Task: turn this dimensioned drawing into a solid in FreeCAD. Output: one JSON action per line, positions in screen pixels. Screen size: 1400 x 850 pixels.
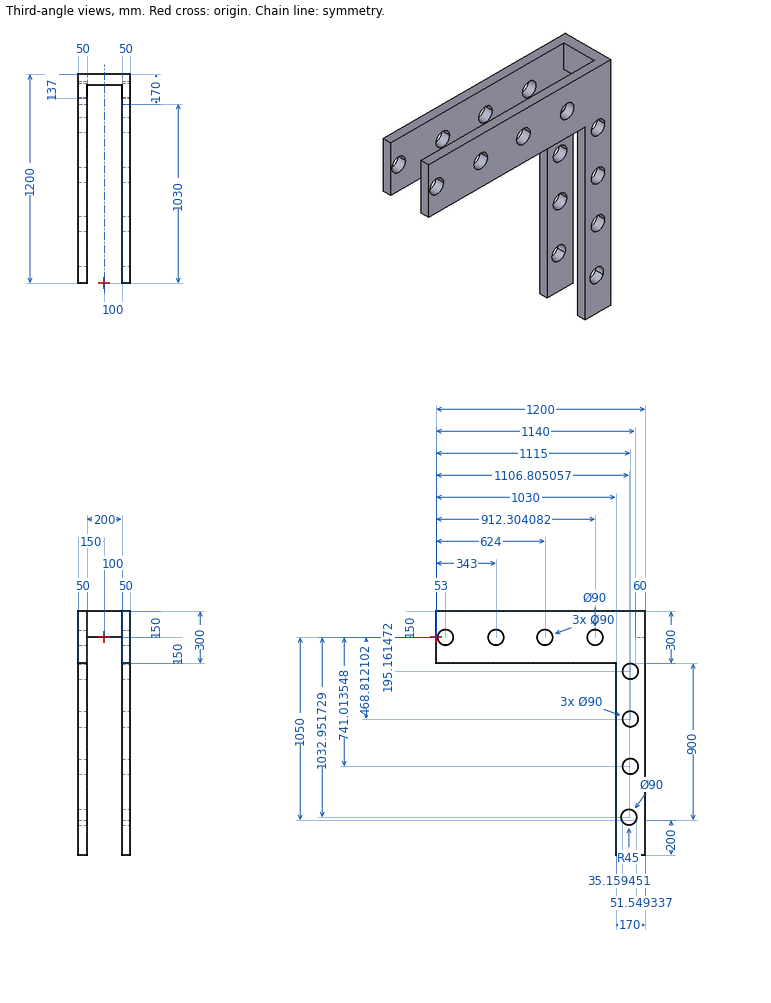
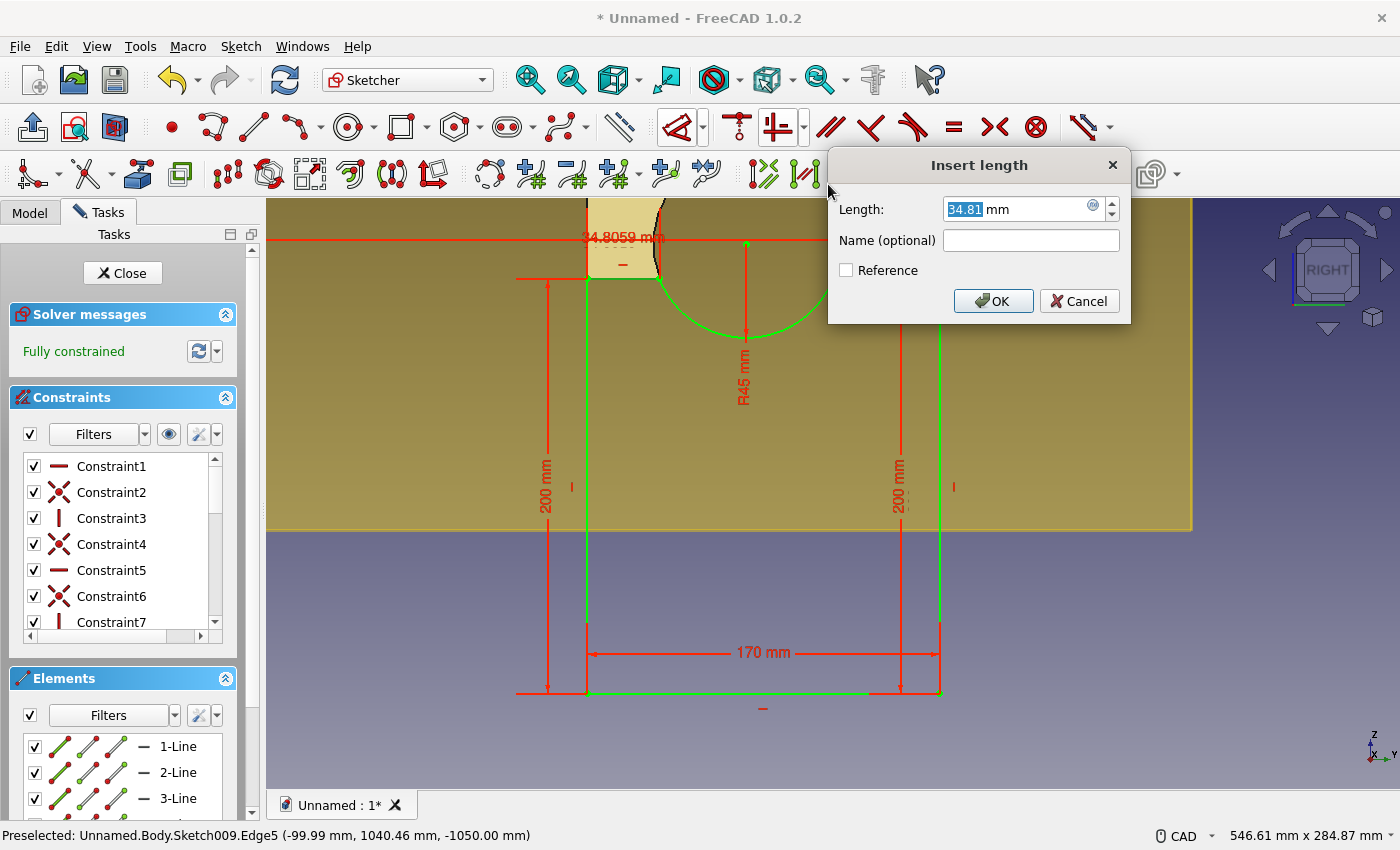
{"action": "type", "text": "35.159451"}
{"action": "key", "text": "Return"}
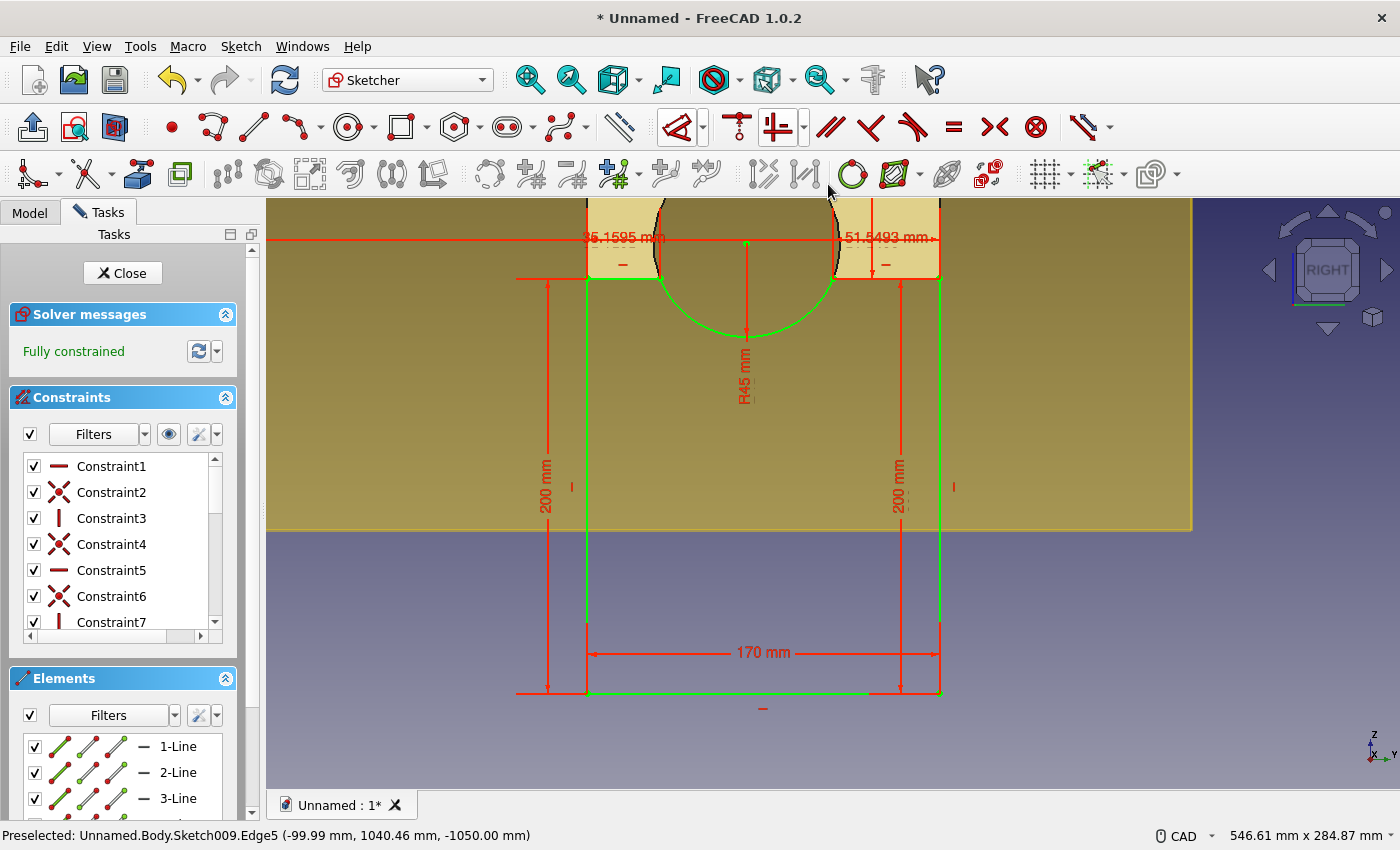
{"action": "left_click", "coordinate": [123, 273]}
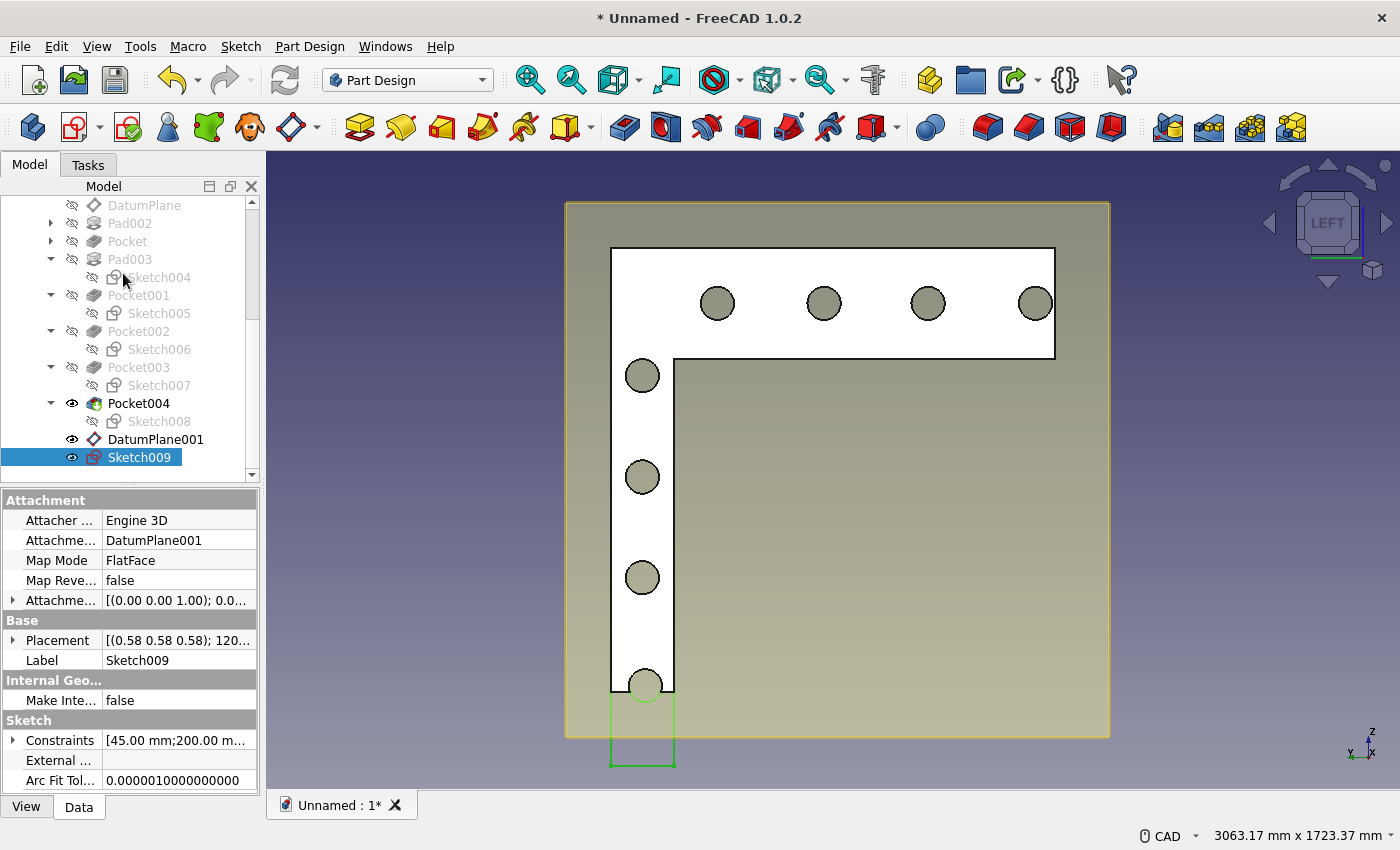
{"action": "left_click", "coordinate": [360, 128]}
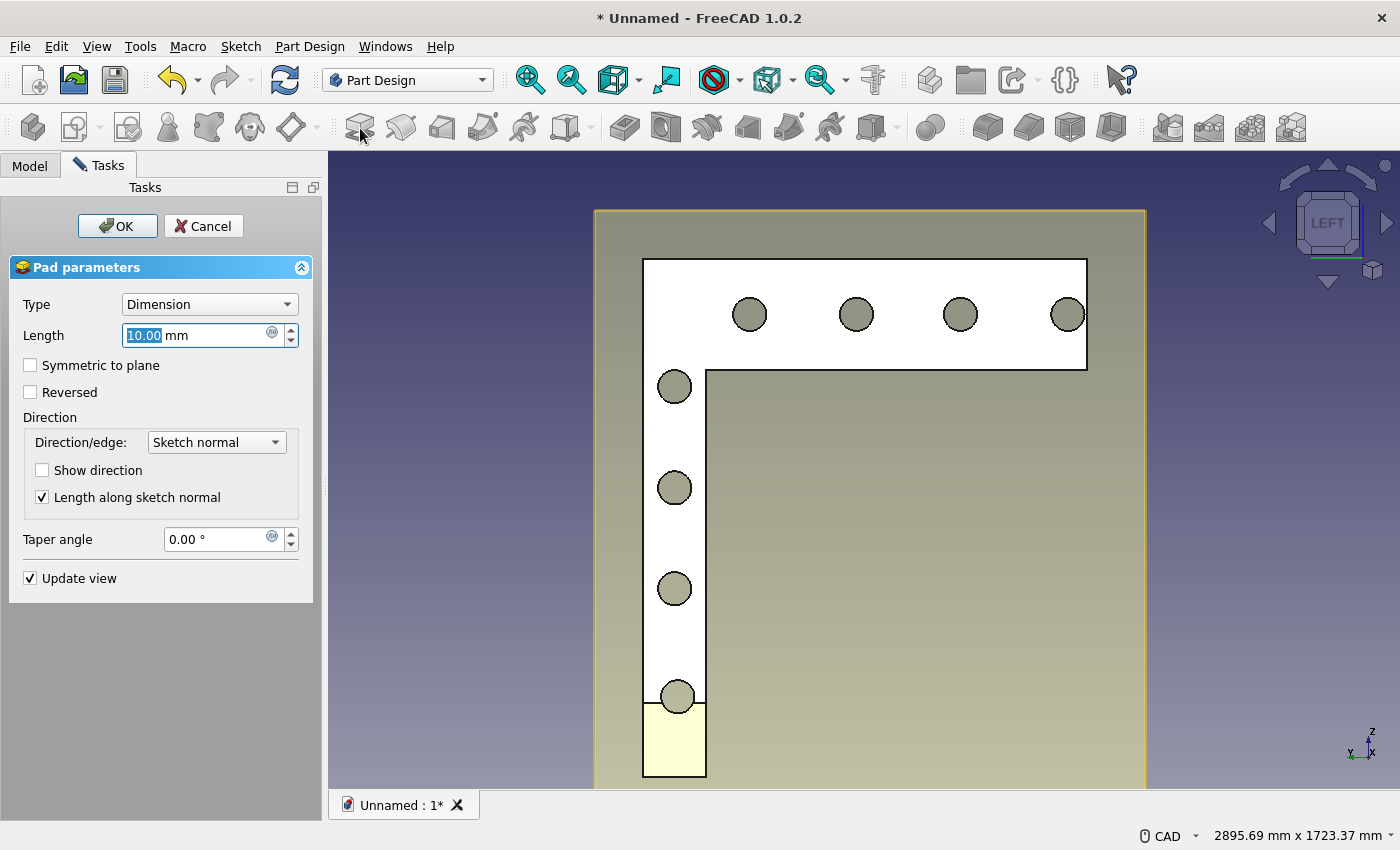
{"action": "type", "text": "50"}
{"action": "key", "text": "Tab"}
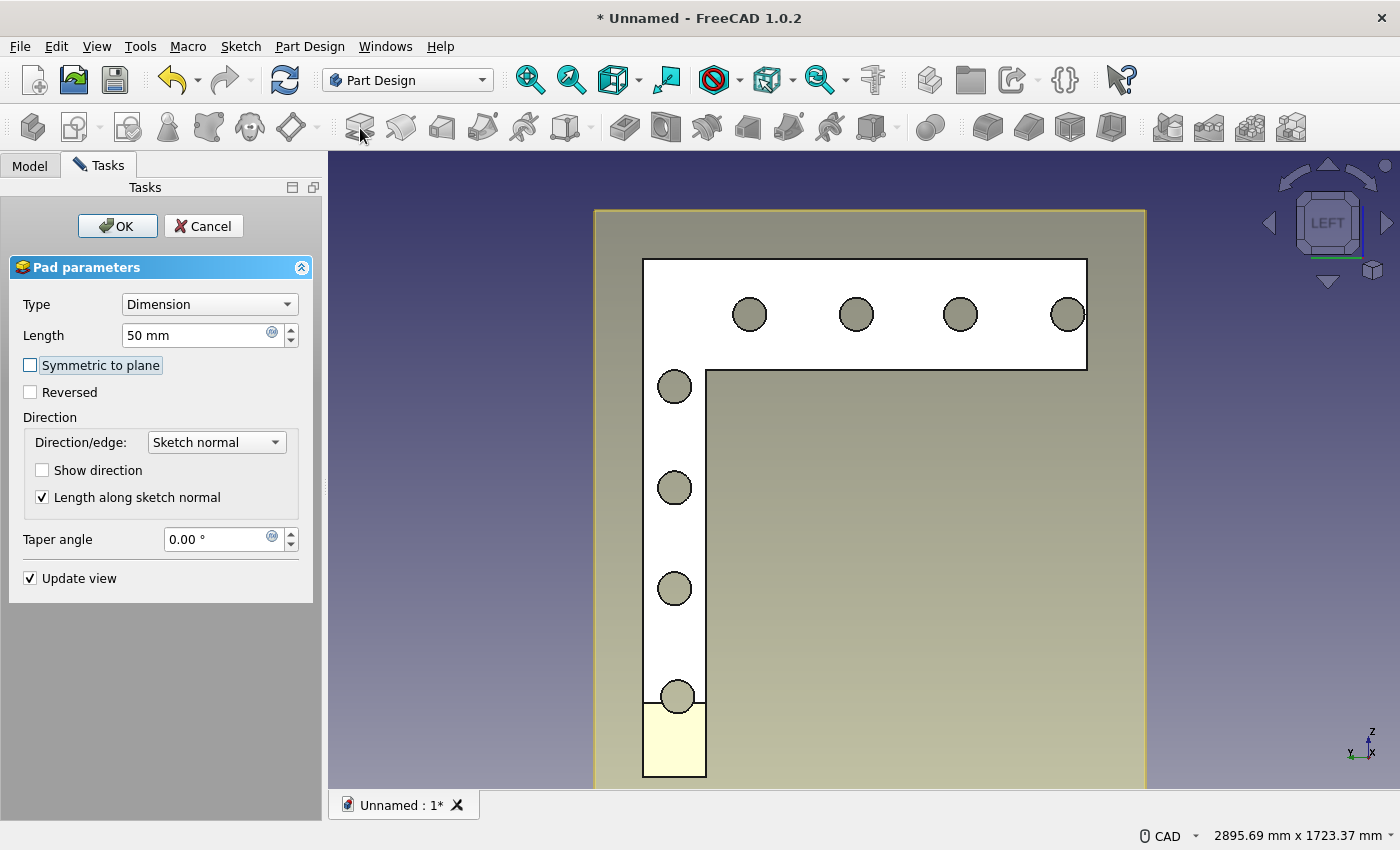
{"action": "left_click", "coordinate": [31, 392]}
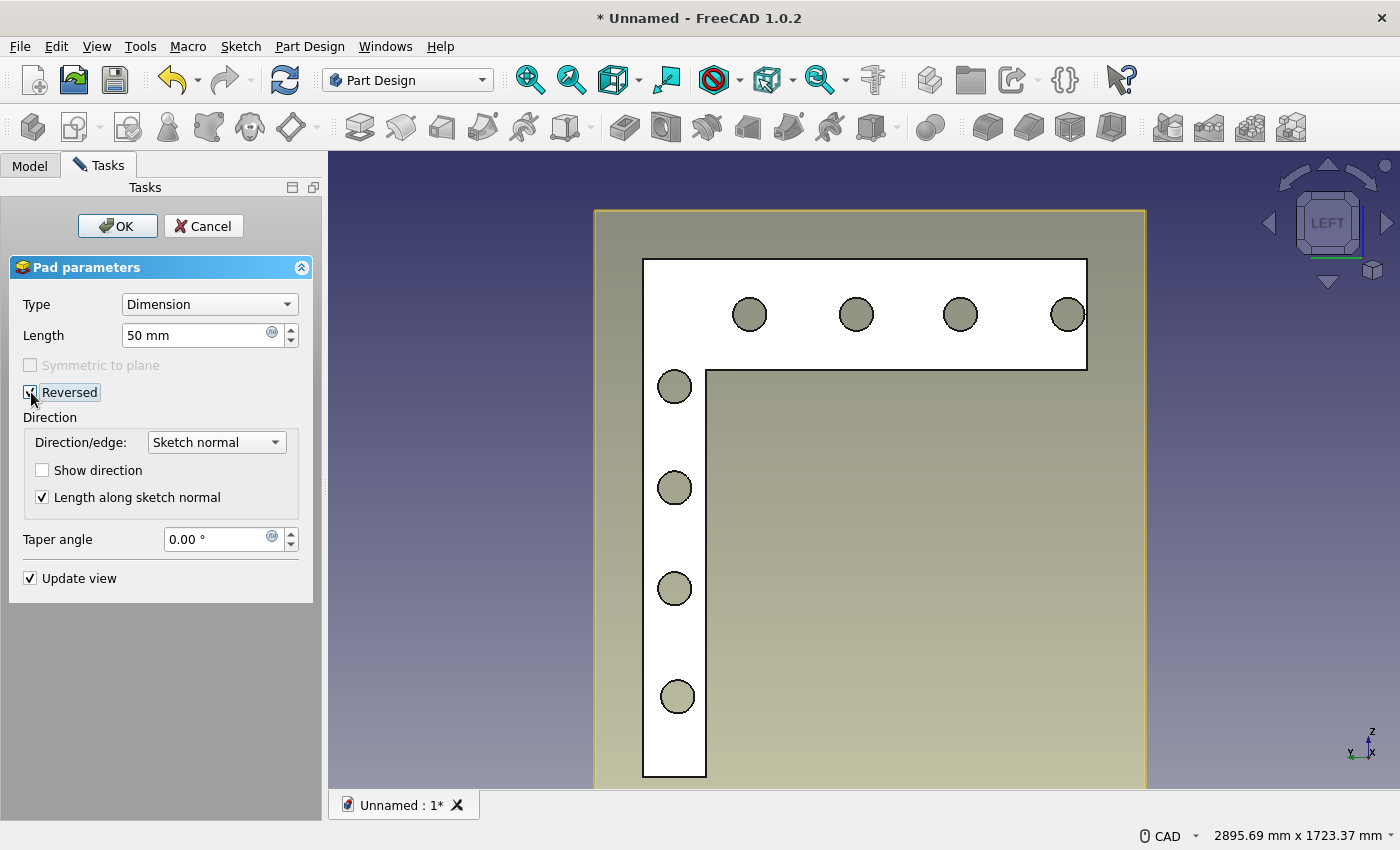
{"action": "left_click", "coordinate": [118, 226]}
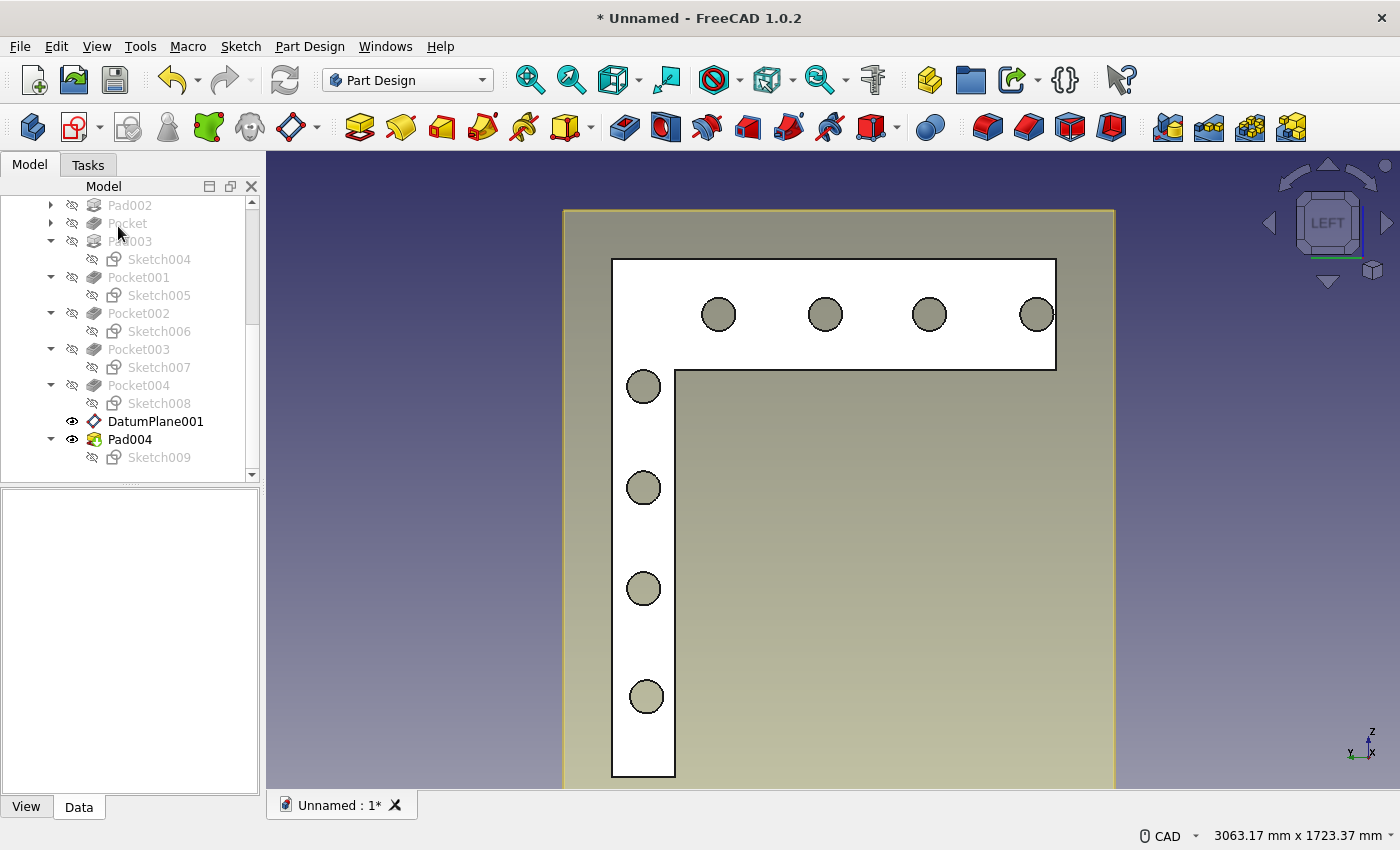
{"action": "left_click", "coordinate": [117, 421]}
{"action": "key", "text": "space"}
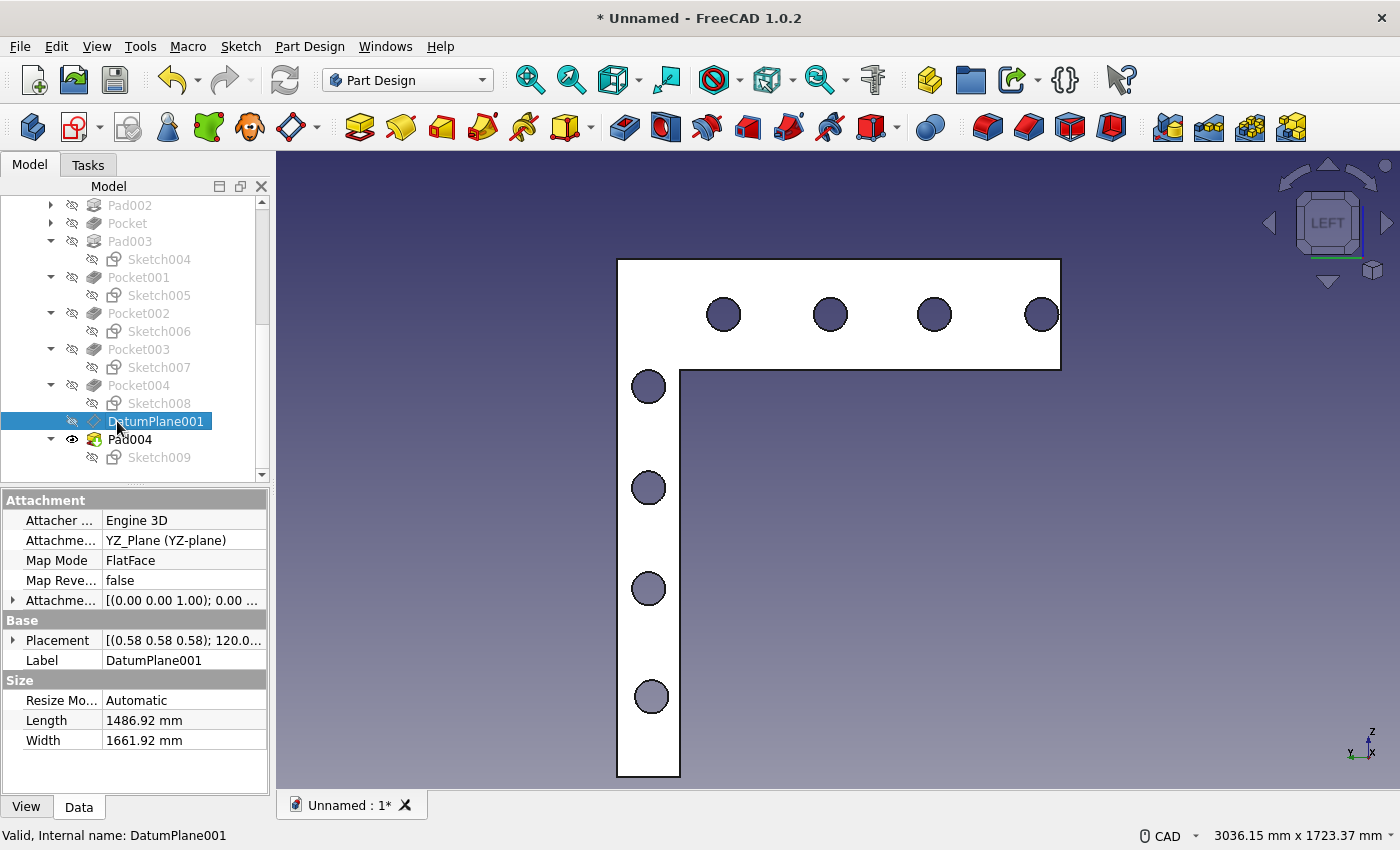
{"action": "key", "text": "0"}